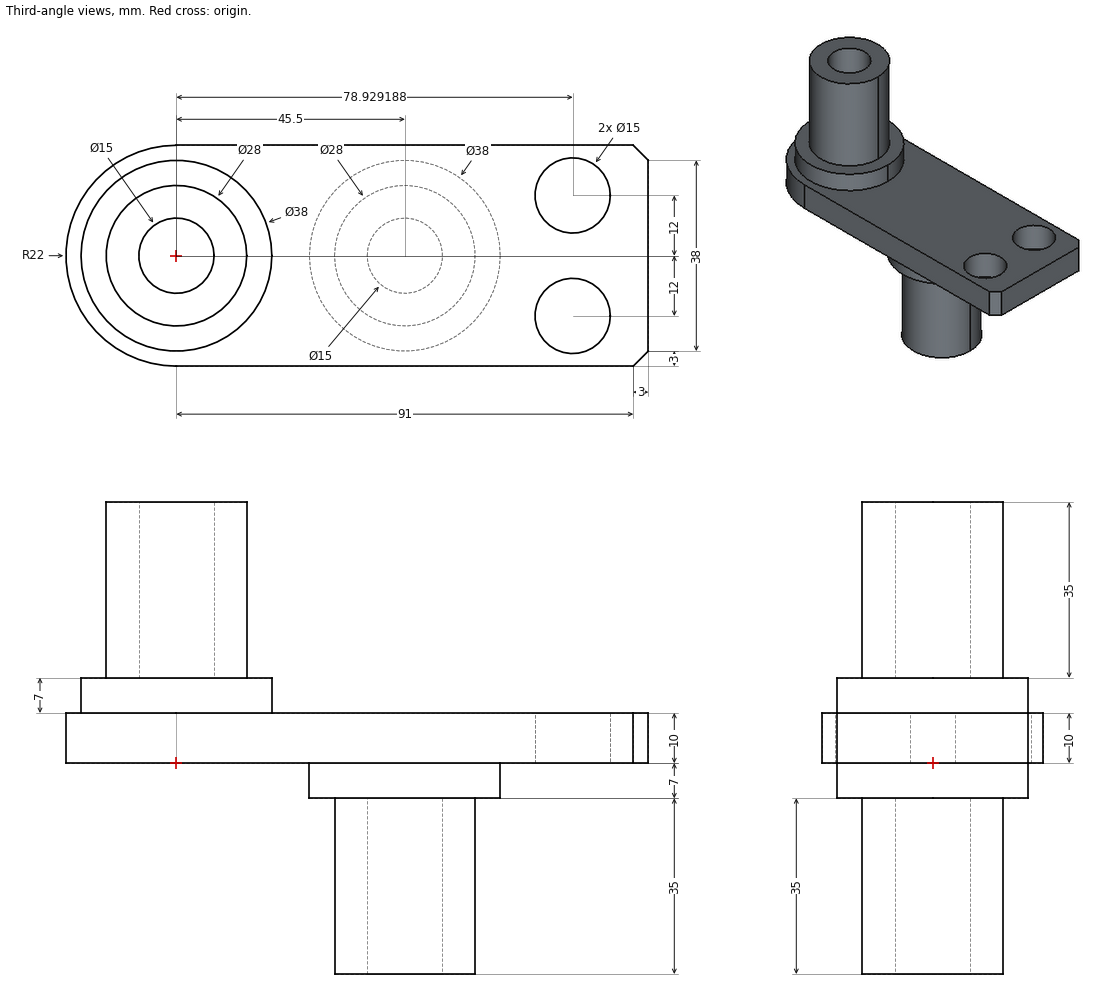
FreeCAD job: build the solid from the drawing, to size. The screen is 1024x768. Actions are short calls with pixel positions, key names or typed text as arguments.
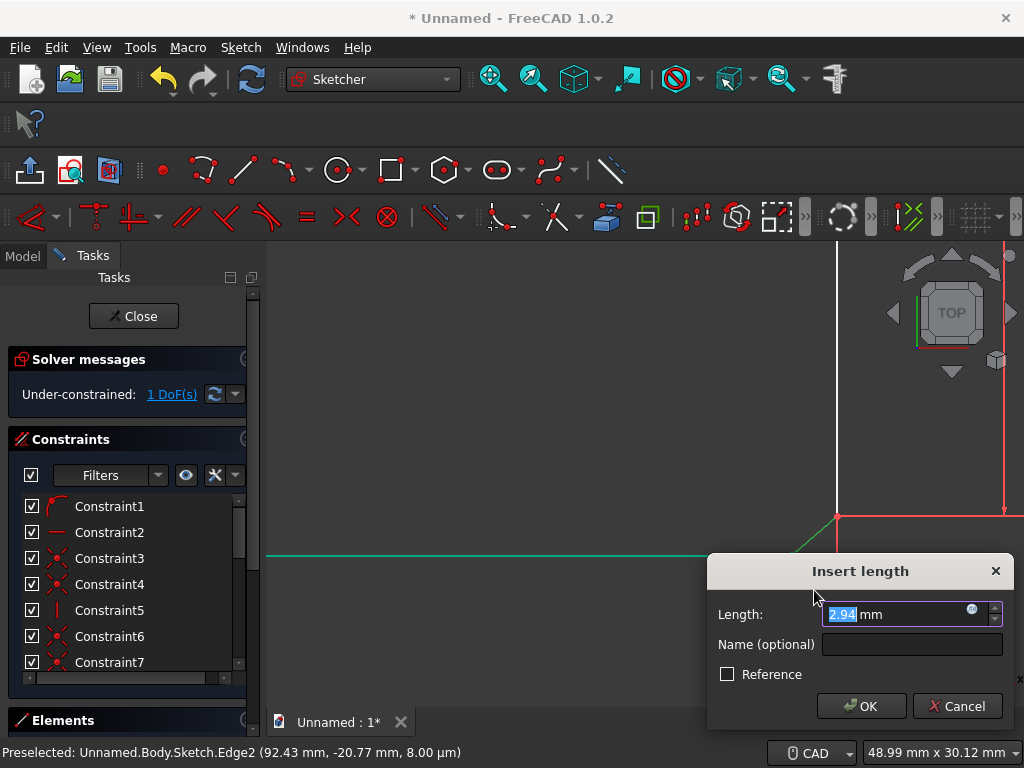
text(3)
key(Return)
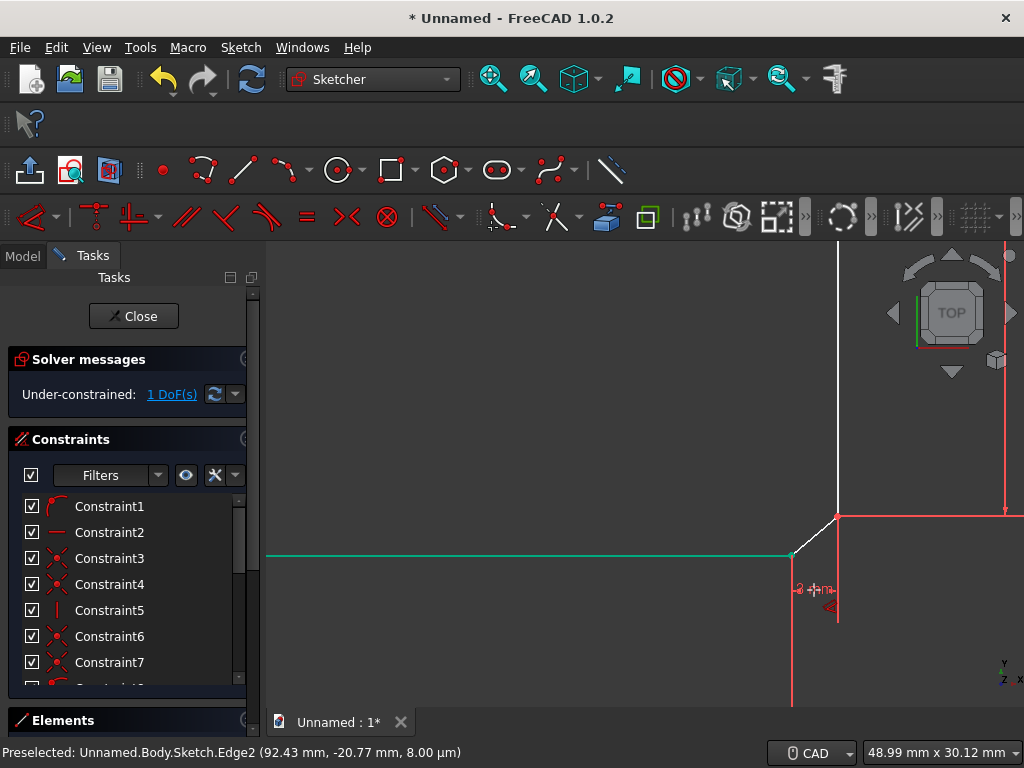
click(805, 544)
click(758, 536)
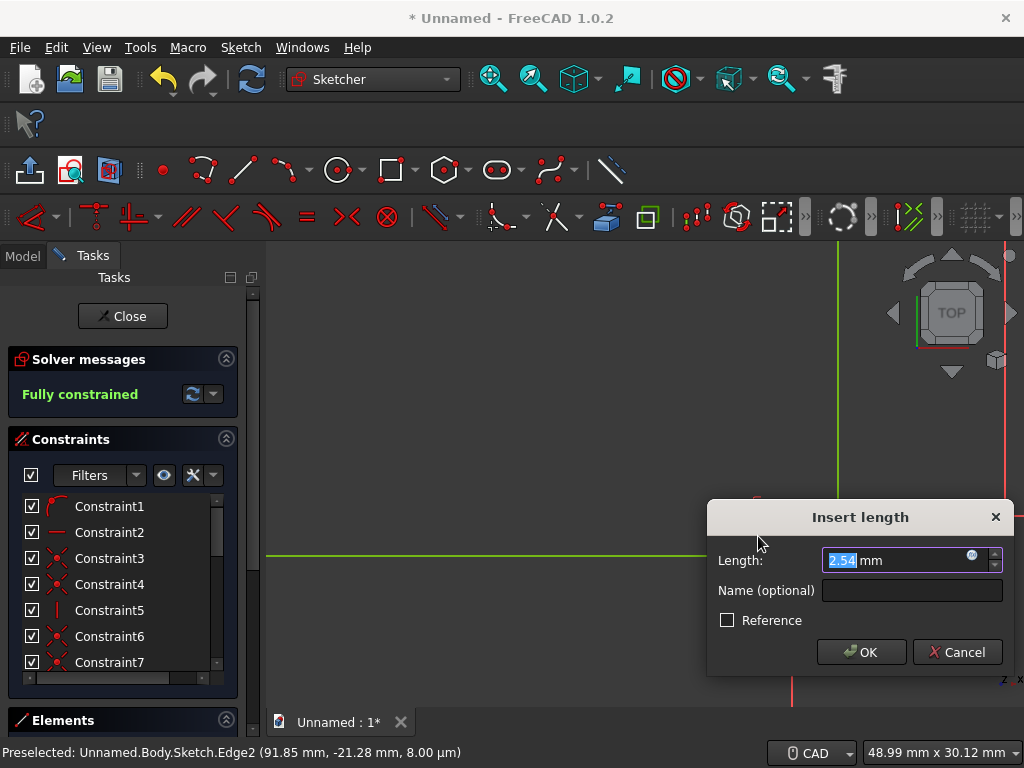
text(3)
key(Return)
key(Escape)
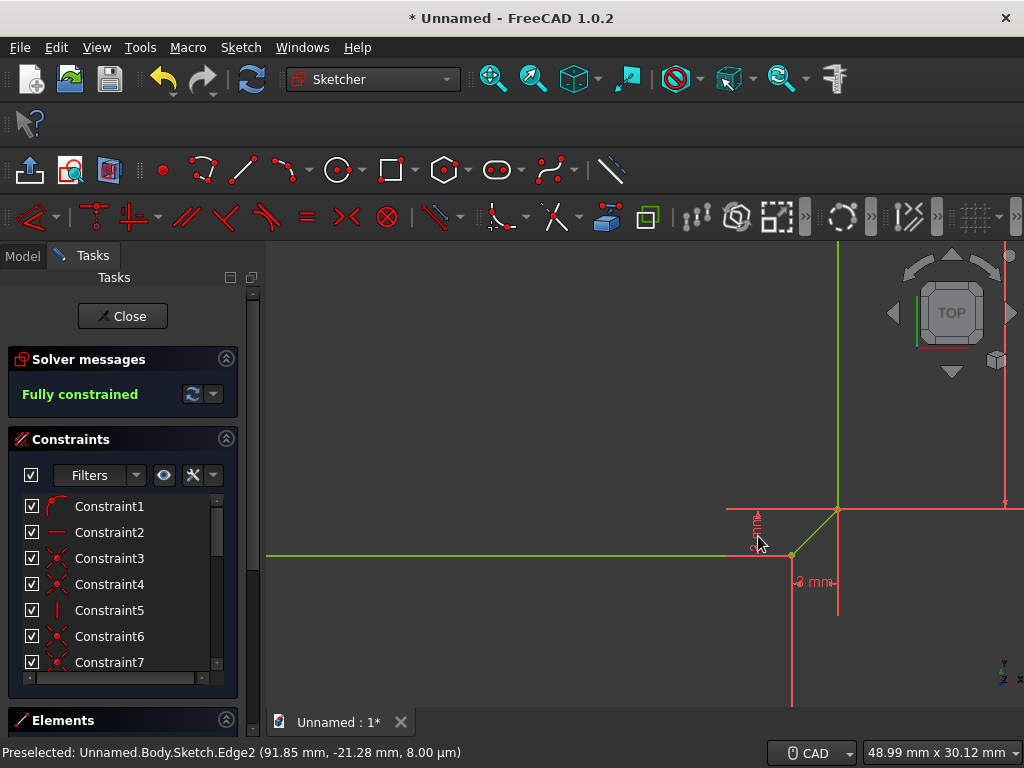
click(123, 316)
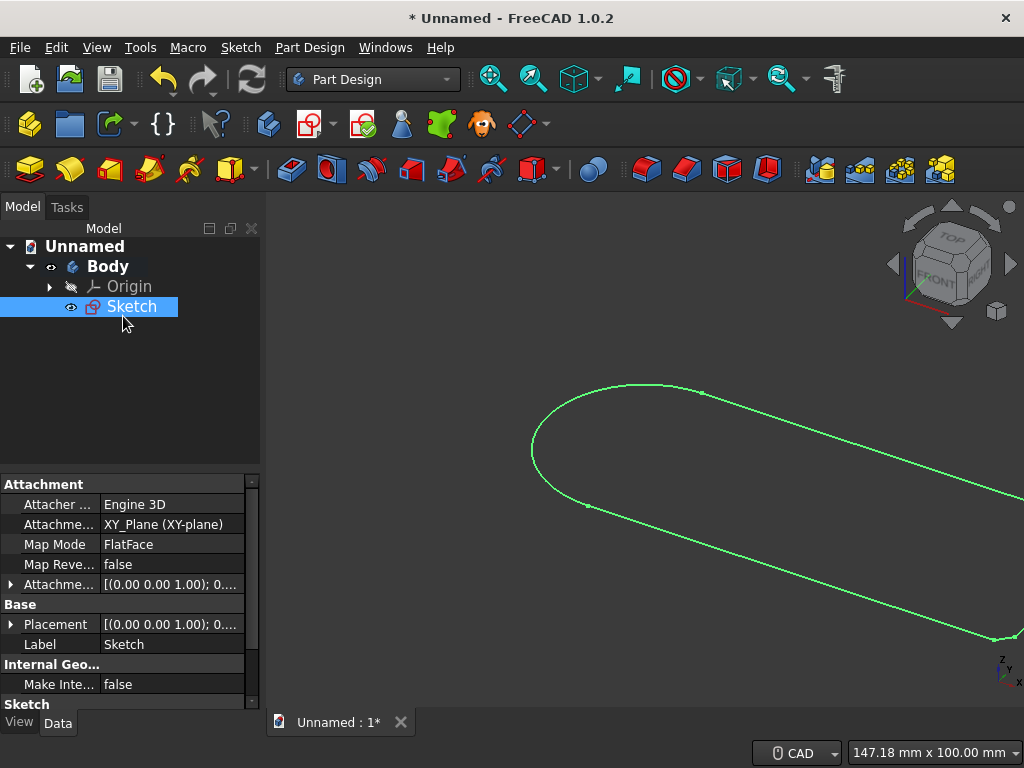
click(30, 170)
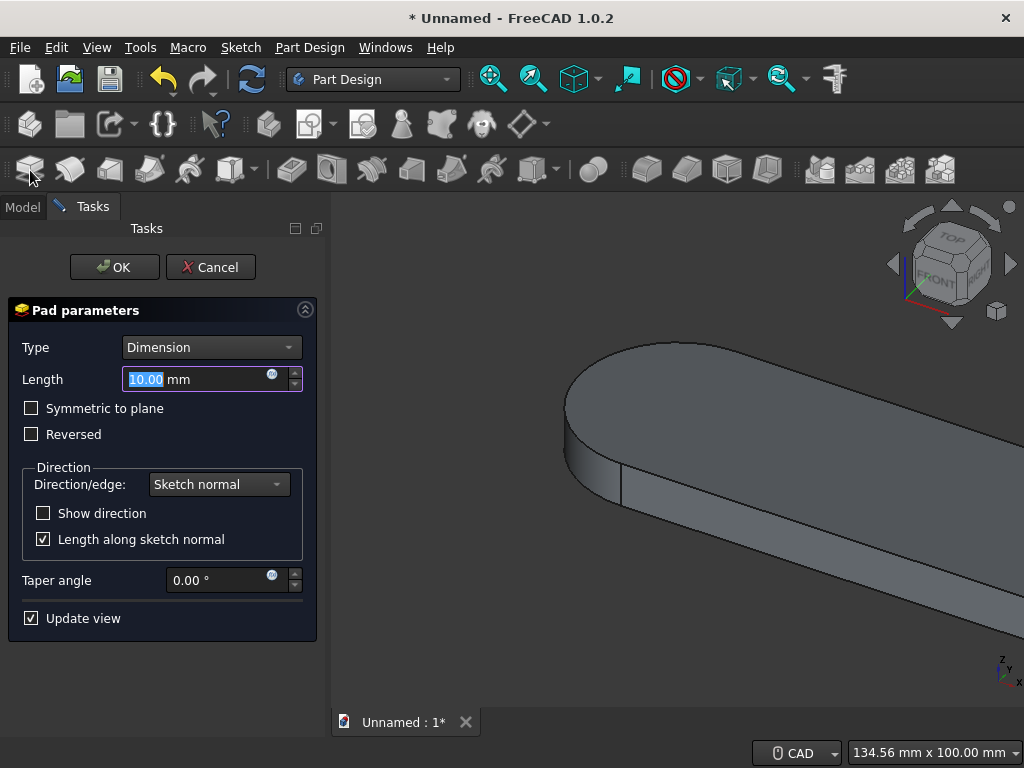
text(10)
key(Tab)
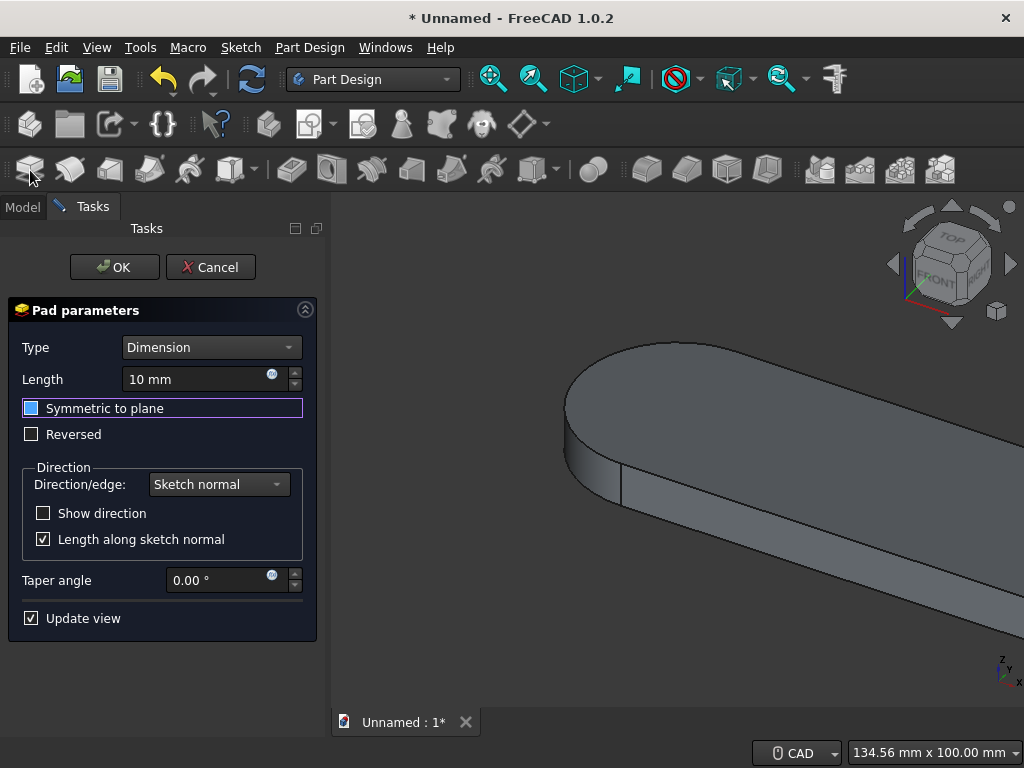
click(115, 267)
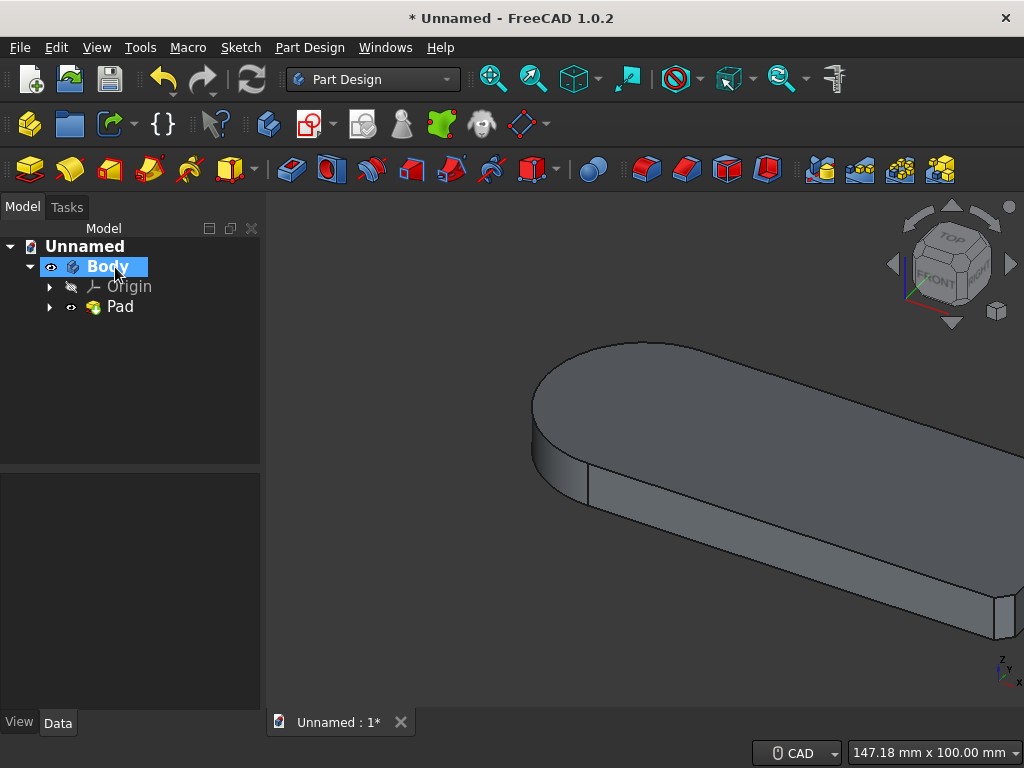
click(494, 80)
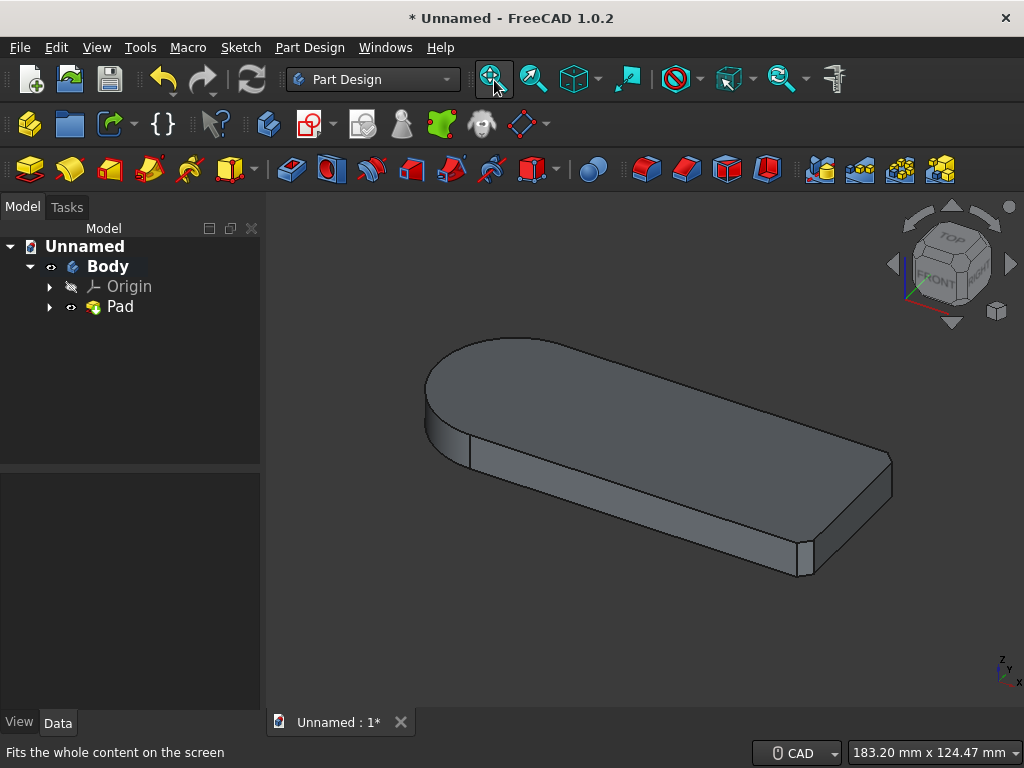
click(764, 471)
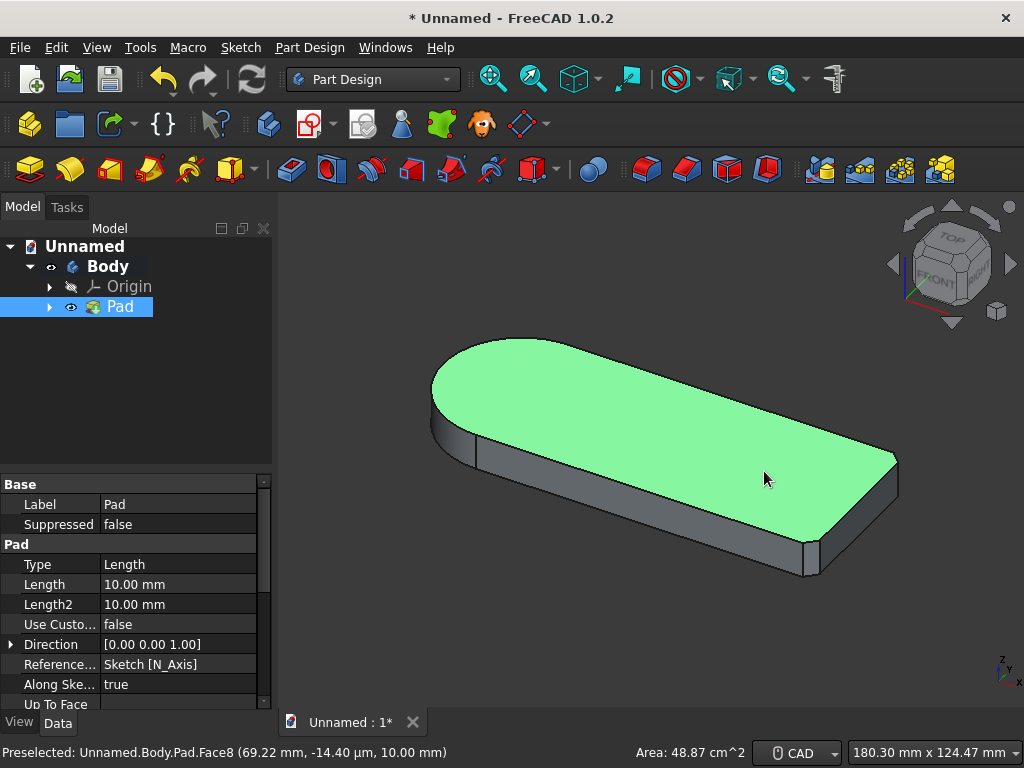
click(310, 124)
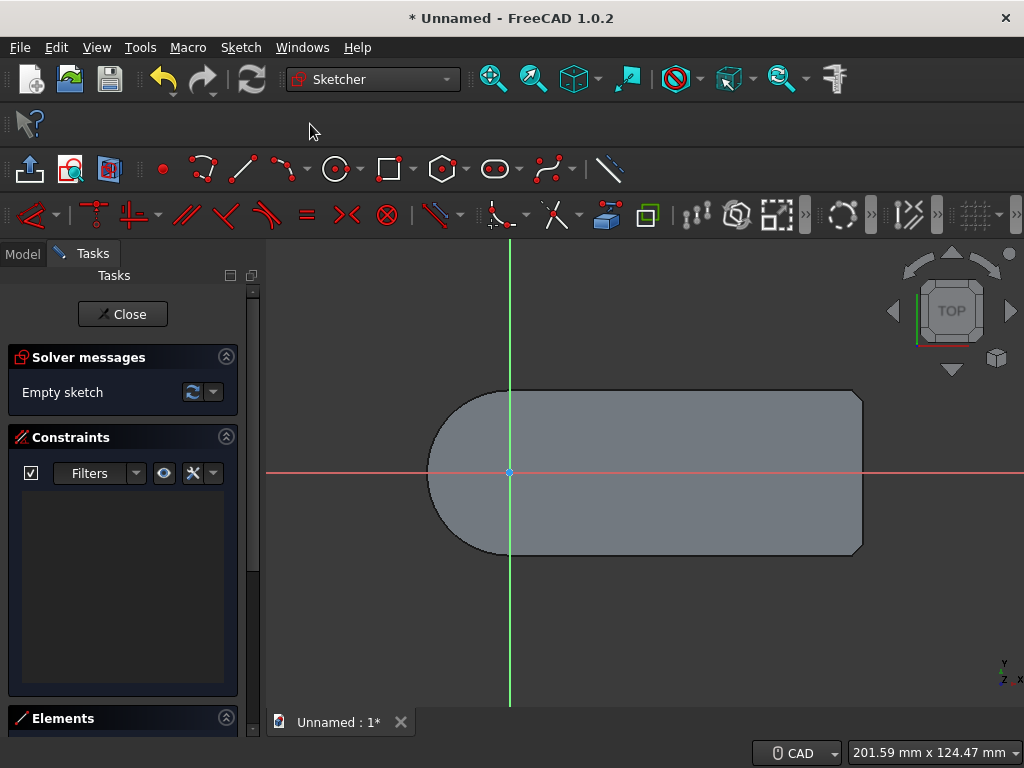
scroll(455, 473, up, 4)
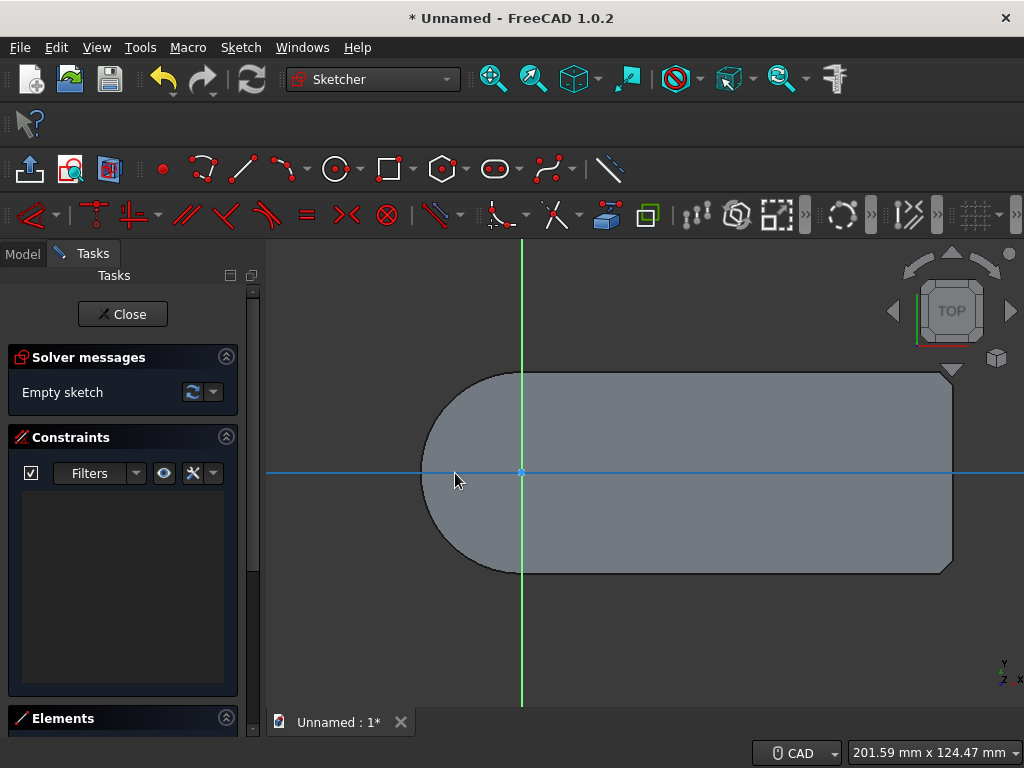
click(336, 170)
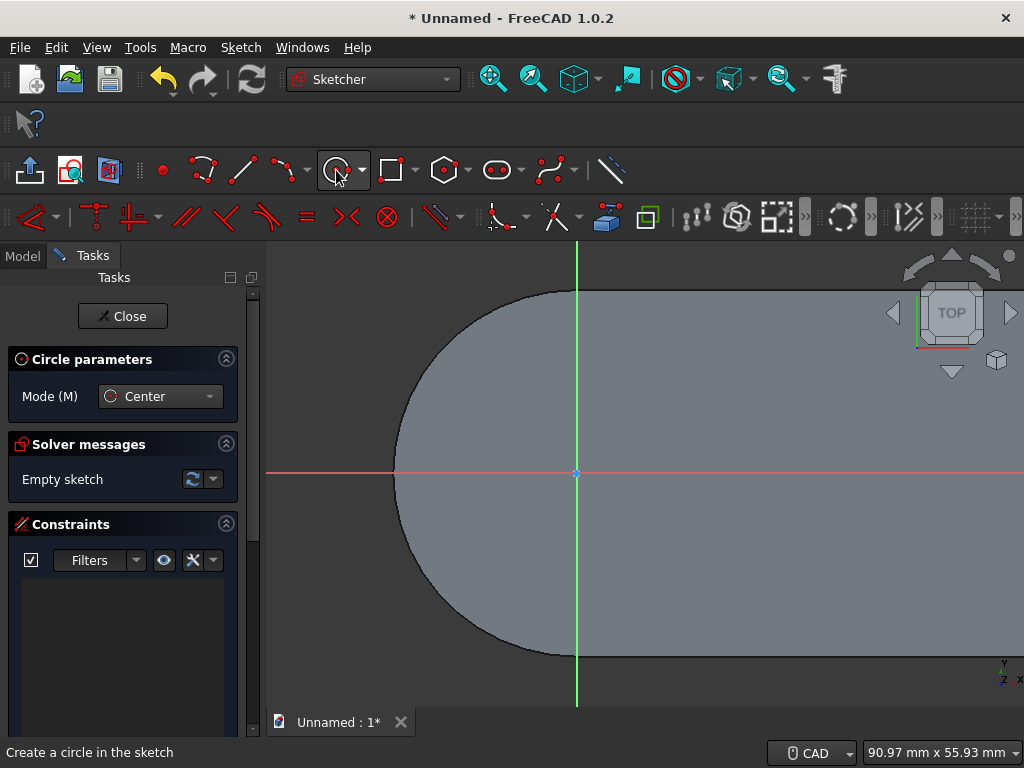
click(577, 473)
move(689, 361)